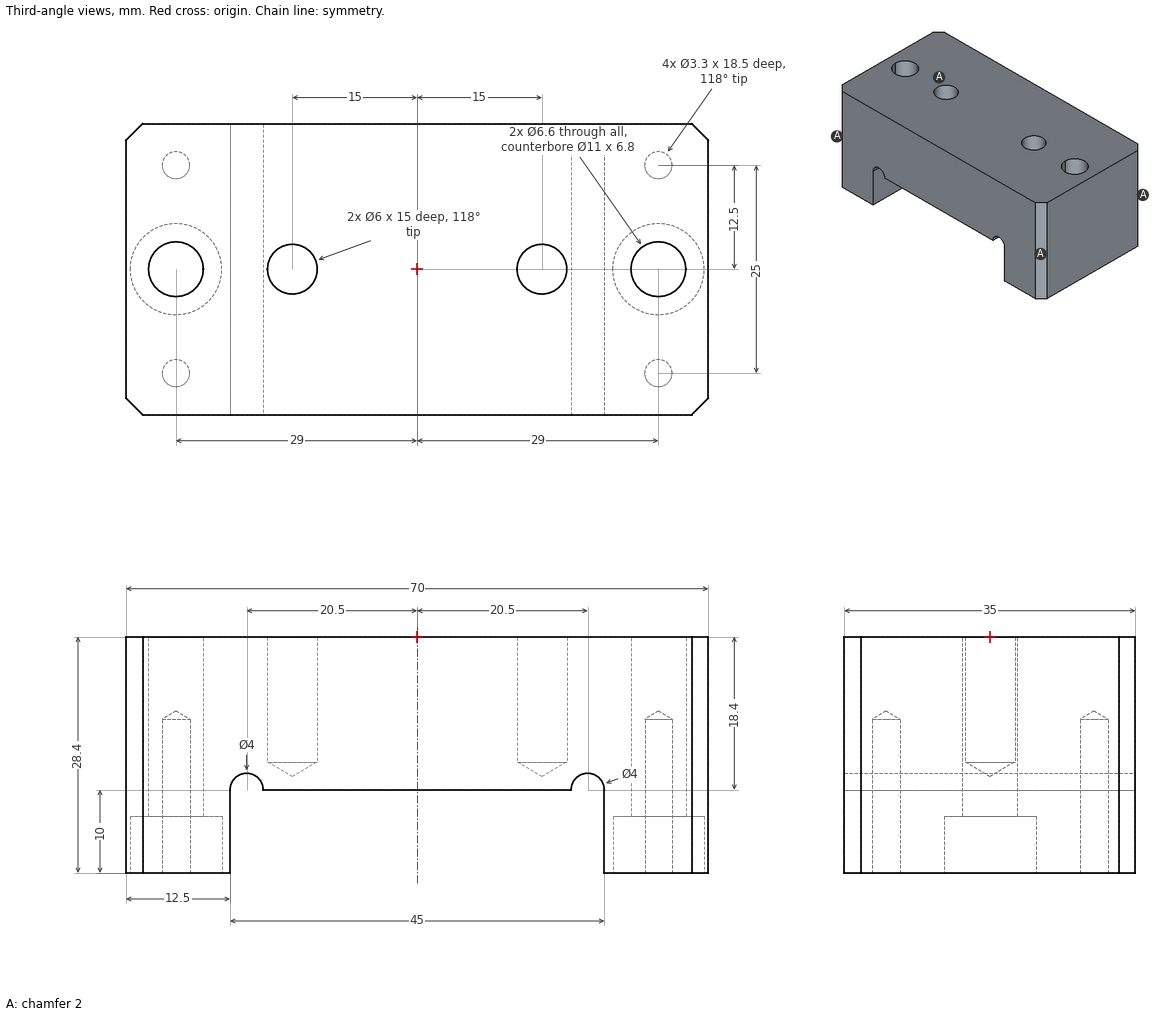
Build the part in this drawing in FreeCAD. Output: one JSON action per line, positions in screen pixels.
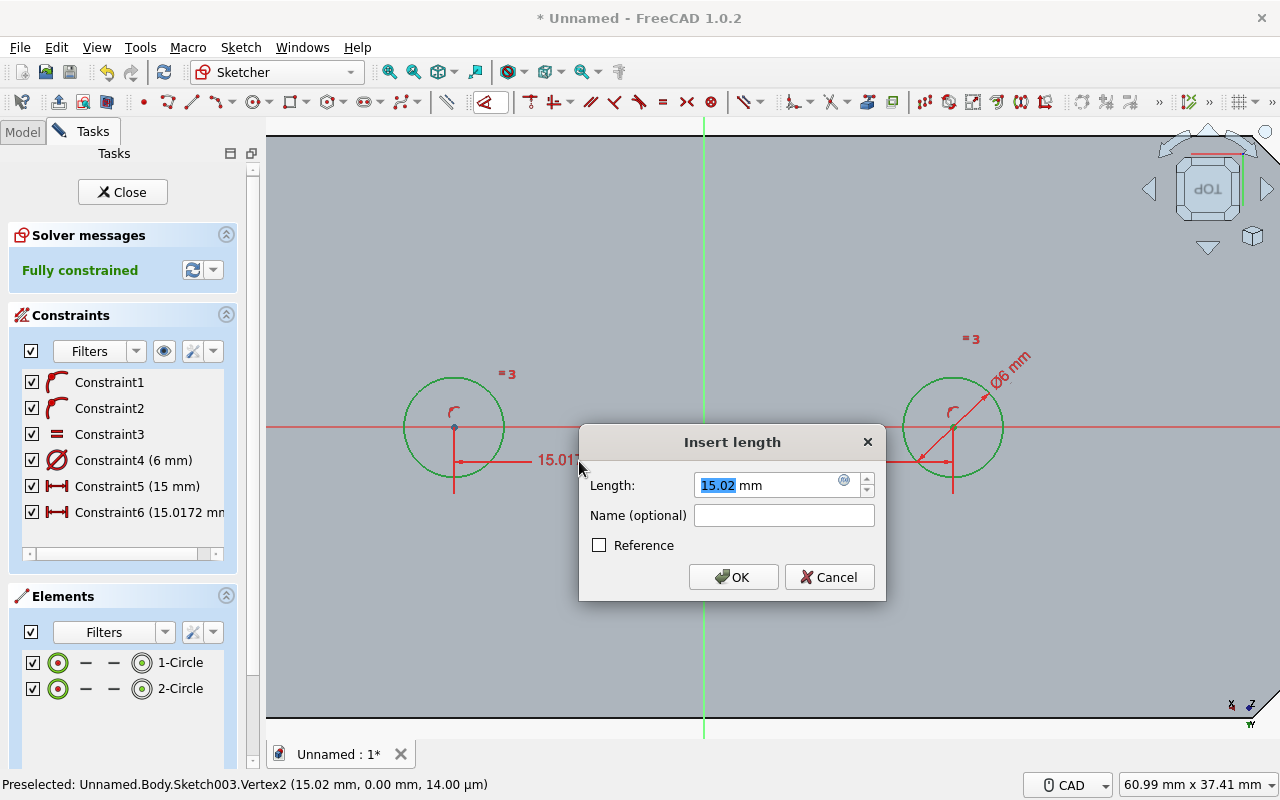
{"action": "type", "text": "15"}
{"action": "key", "text": "Return"}
{"action": "key", "text": "Escape"}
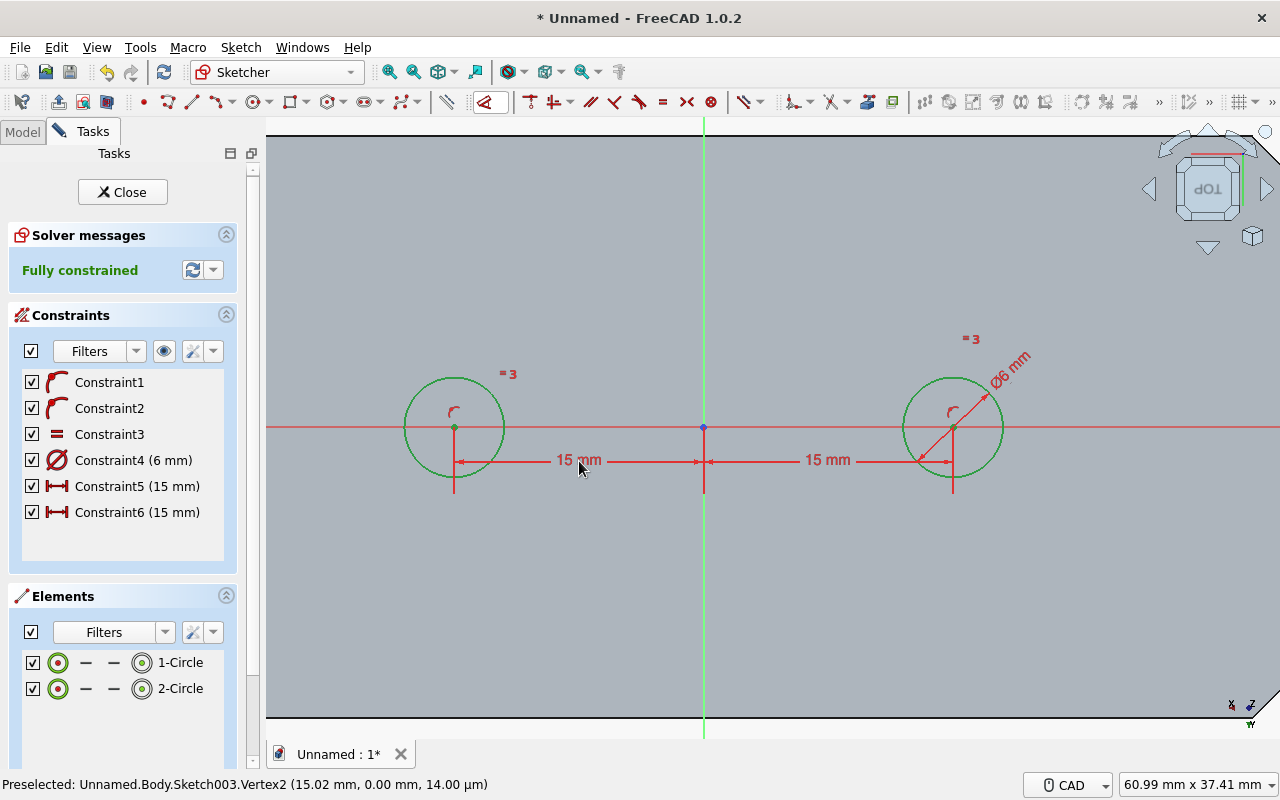
{"action": "left_click", "coordinate": [123, 192]}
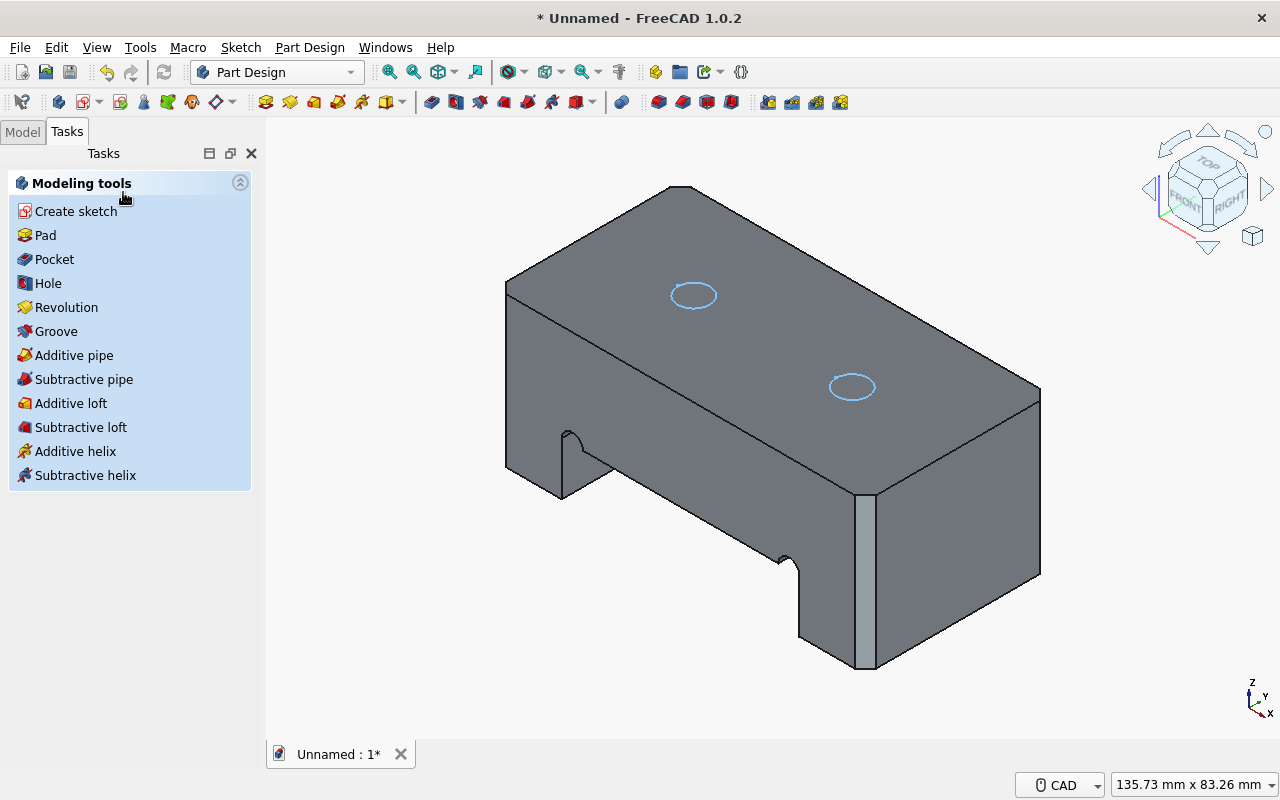
{"action": "left_click", "coordinate": [456, 102]}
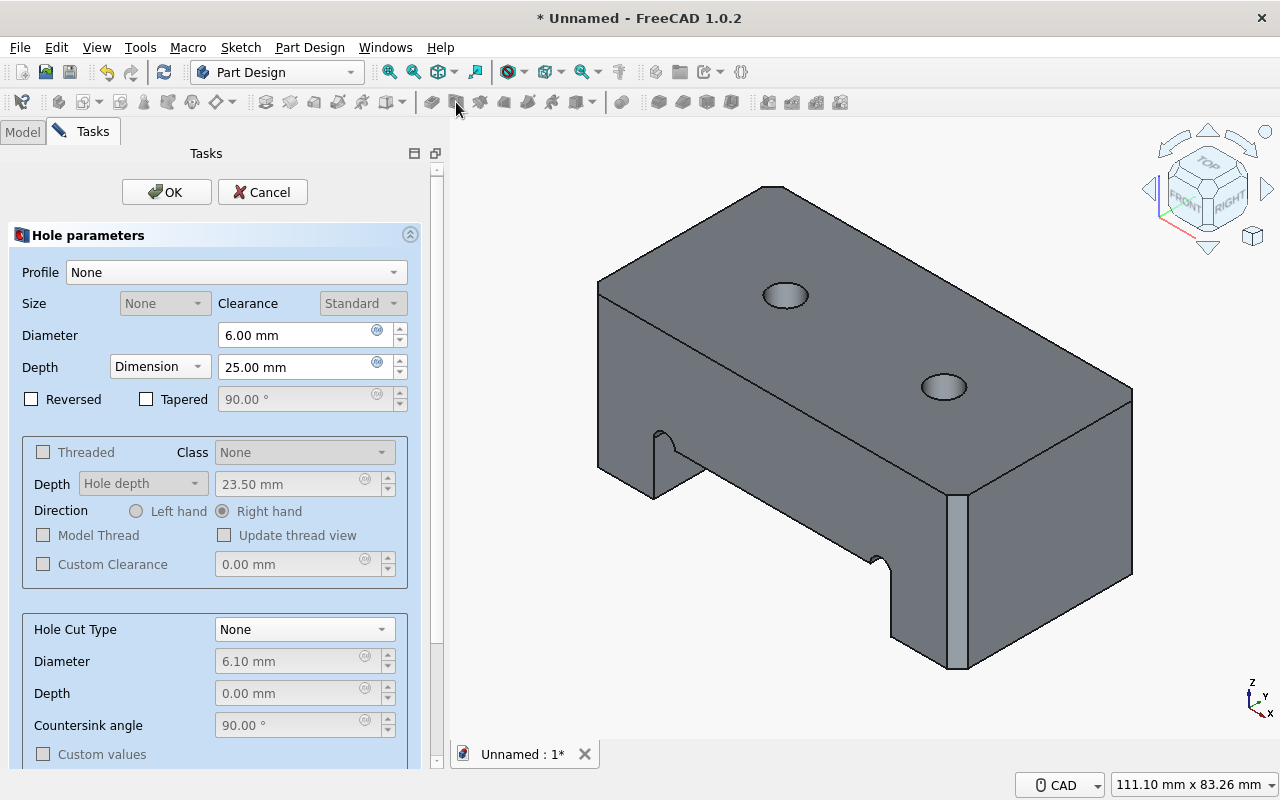
{"action": "triple_click", "coordinate": [305, 335]}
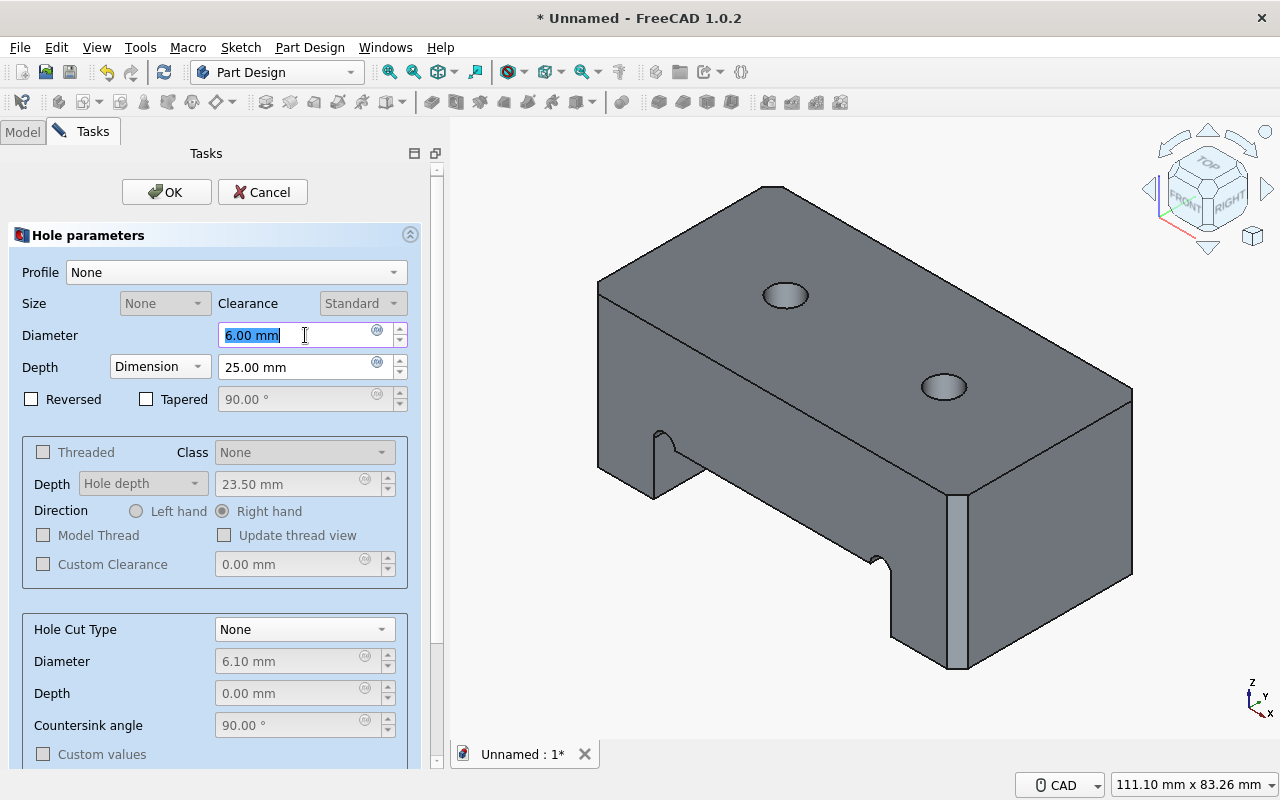
{"action": "type", "text": "6"}
{"action": "key", "text": "Tab"}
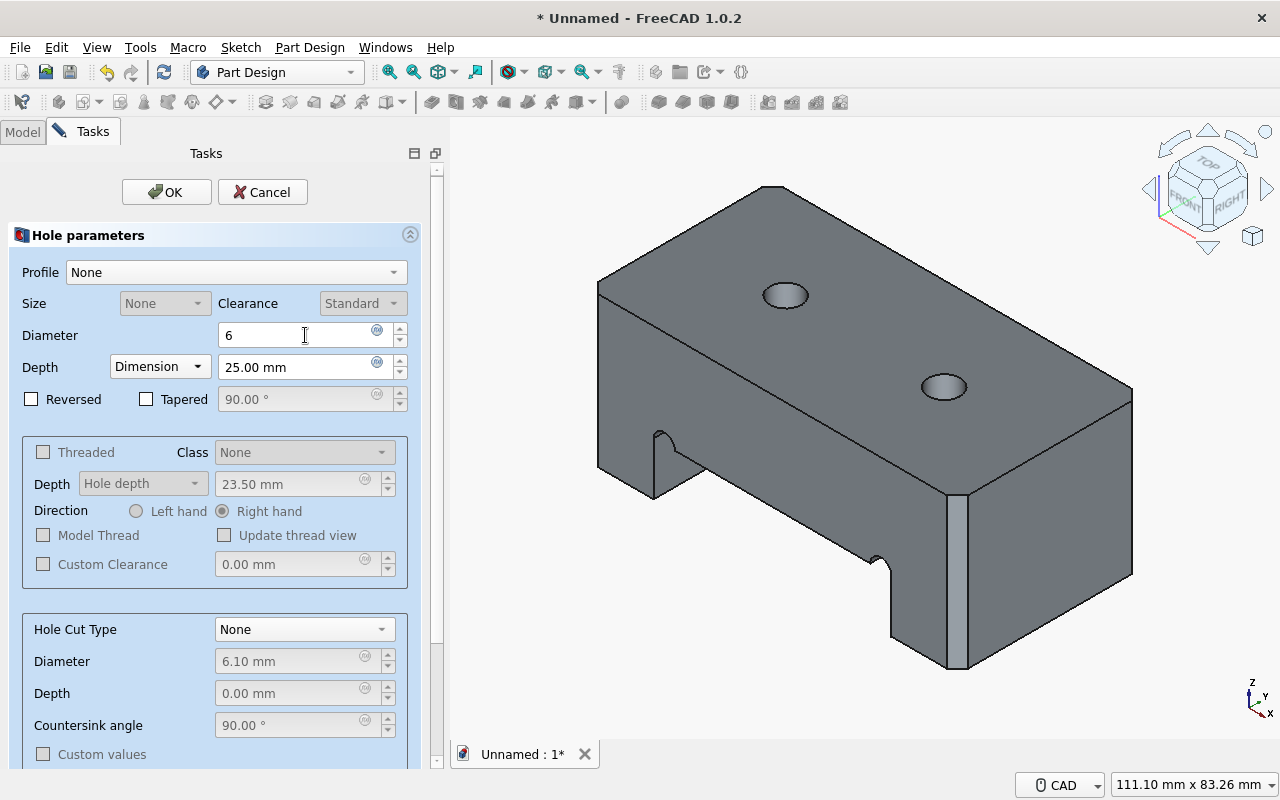
{"action": "triple_click", "coordinate": [305, 367]}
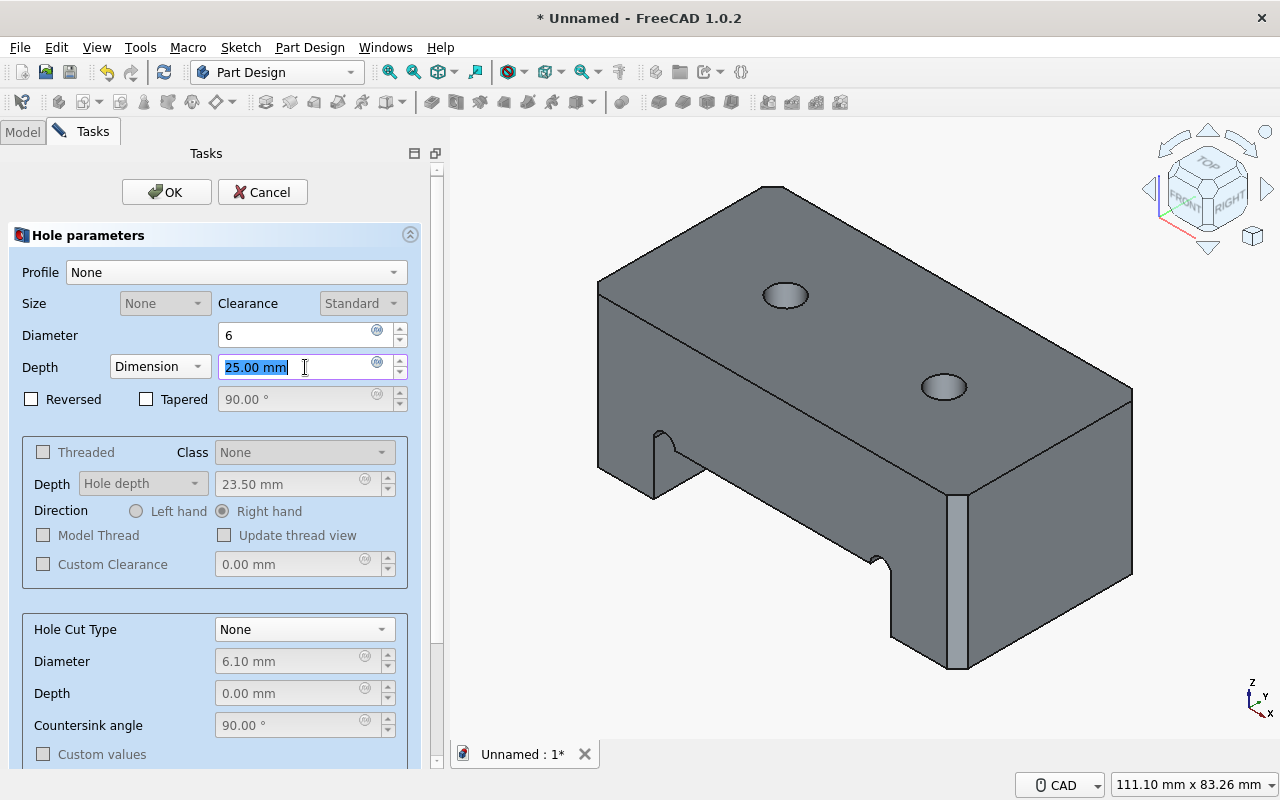
{"action": "type", "text": "15"}
{"action": "key", "text": "Tab"}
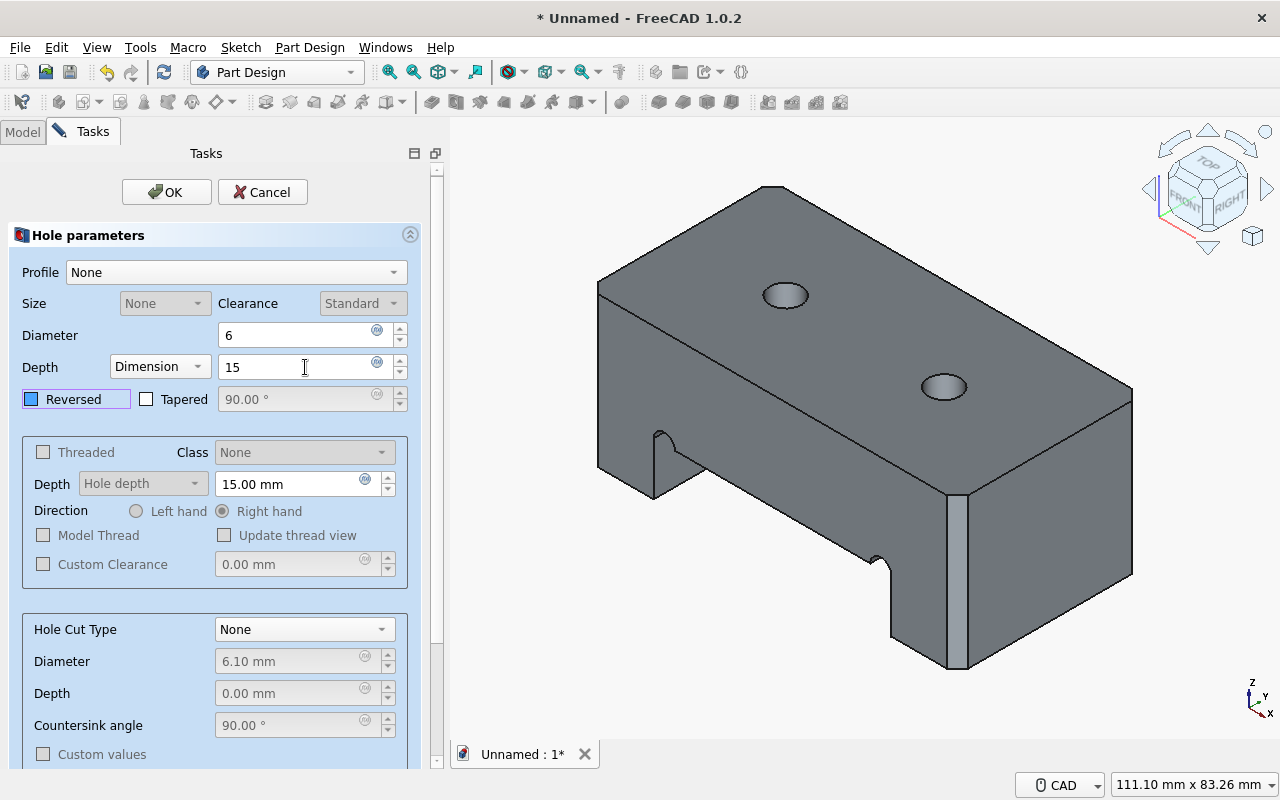
{"action": "left_click", "coordinate": [167, 192]}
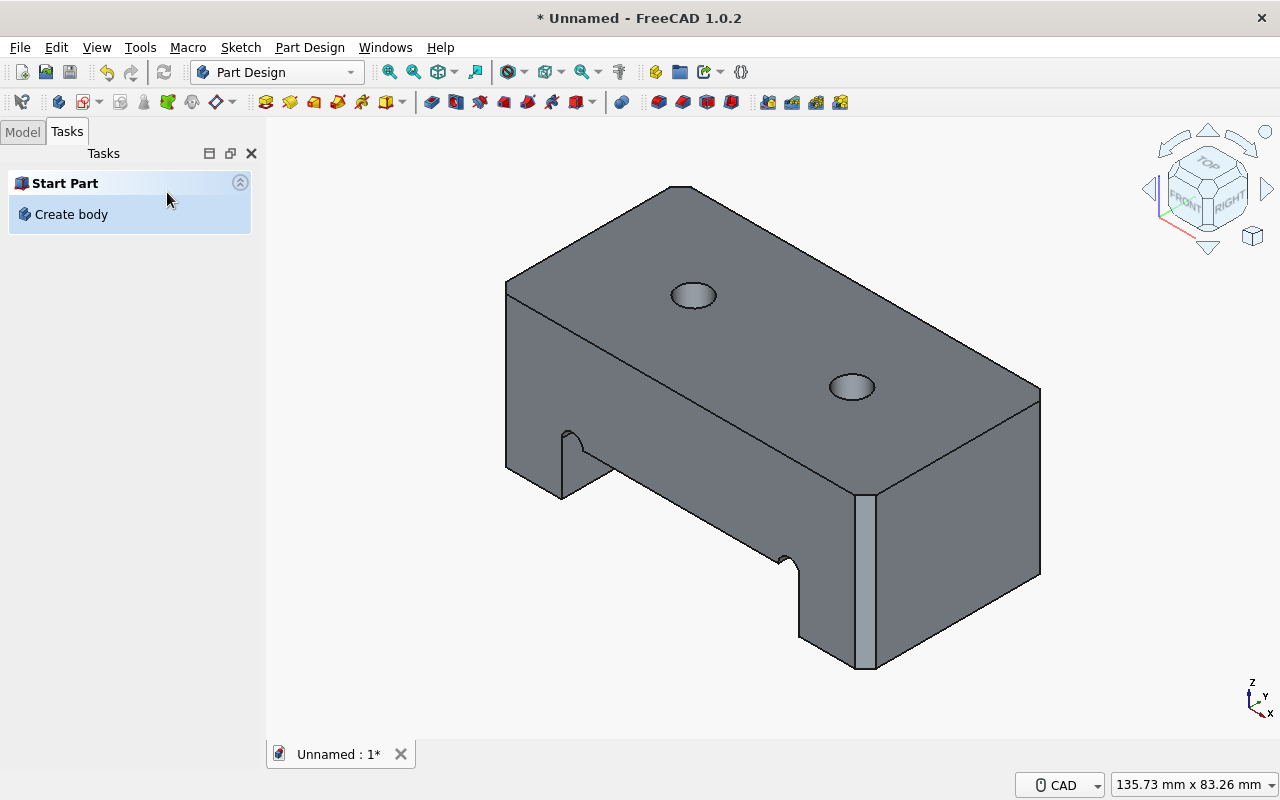
{"action": "key", "text": "5"}